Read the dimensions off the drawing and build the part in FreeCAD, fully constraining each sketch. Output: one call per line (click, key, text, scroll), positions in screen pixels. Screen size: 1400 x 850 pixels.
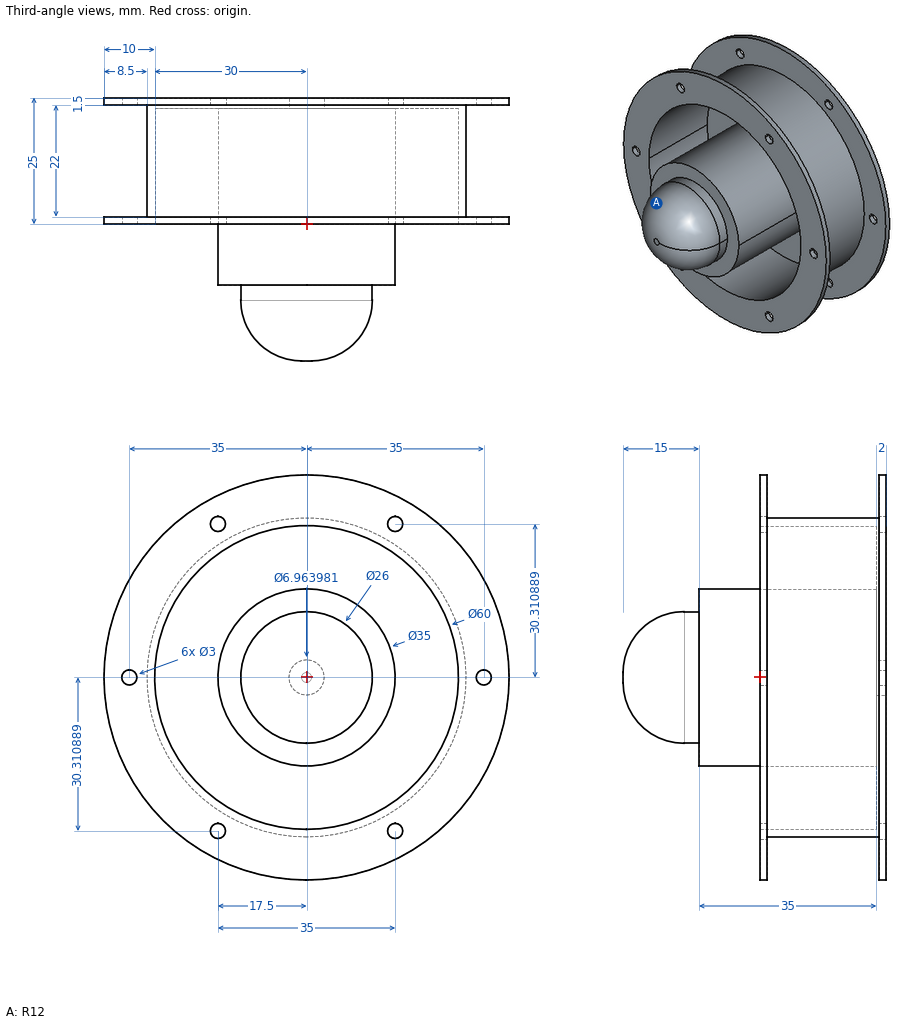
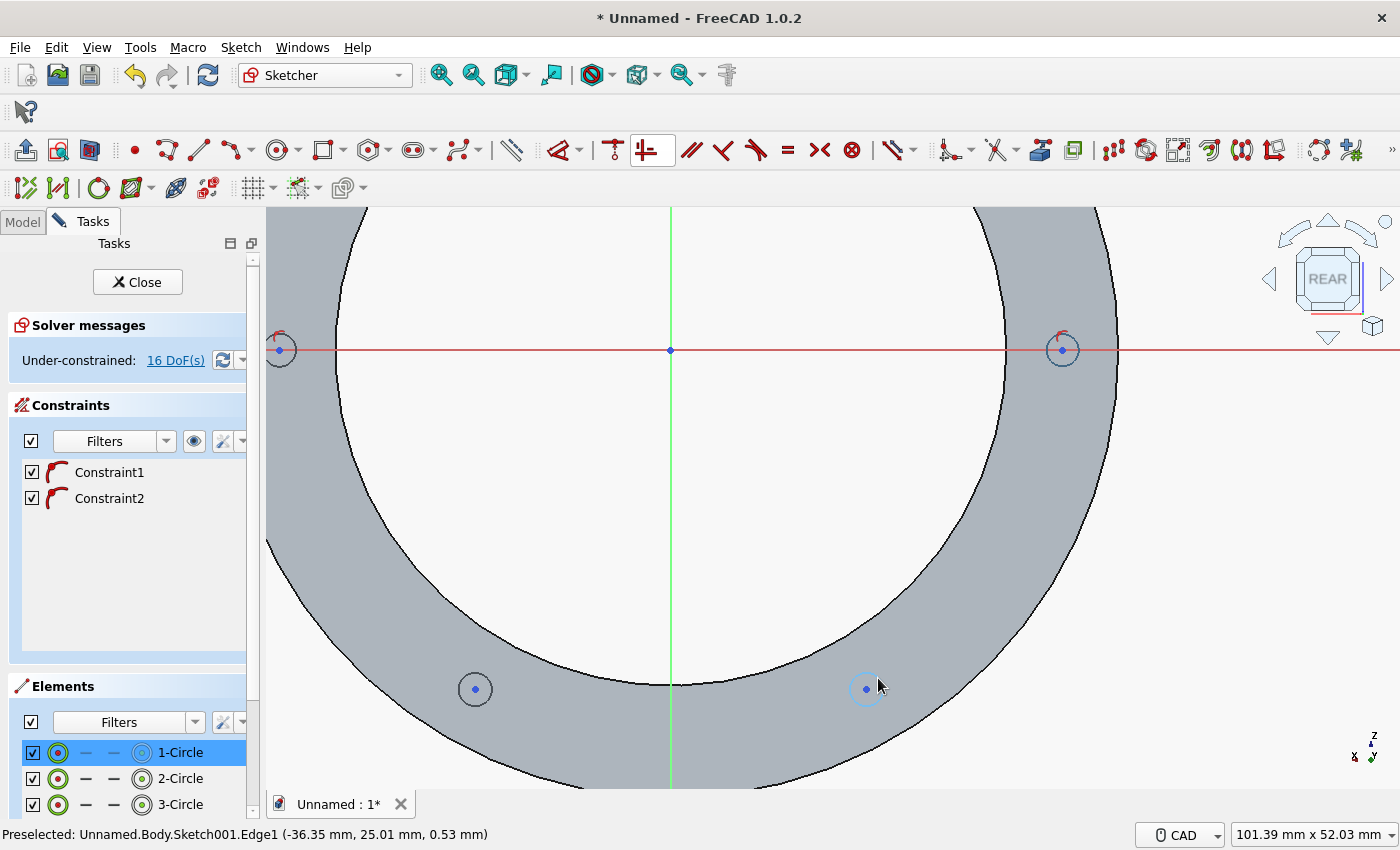
click(878, 678)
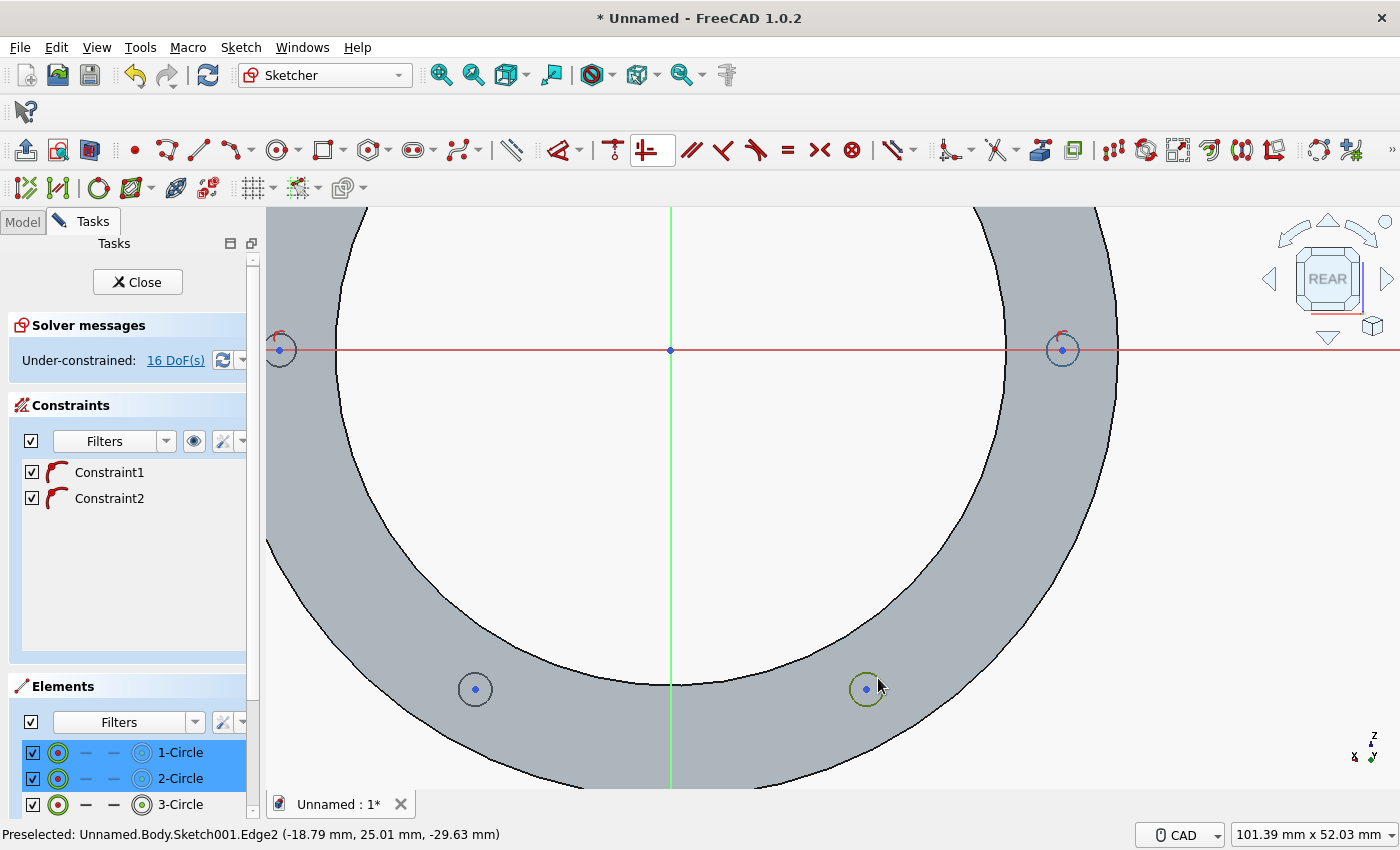
click(487, 678)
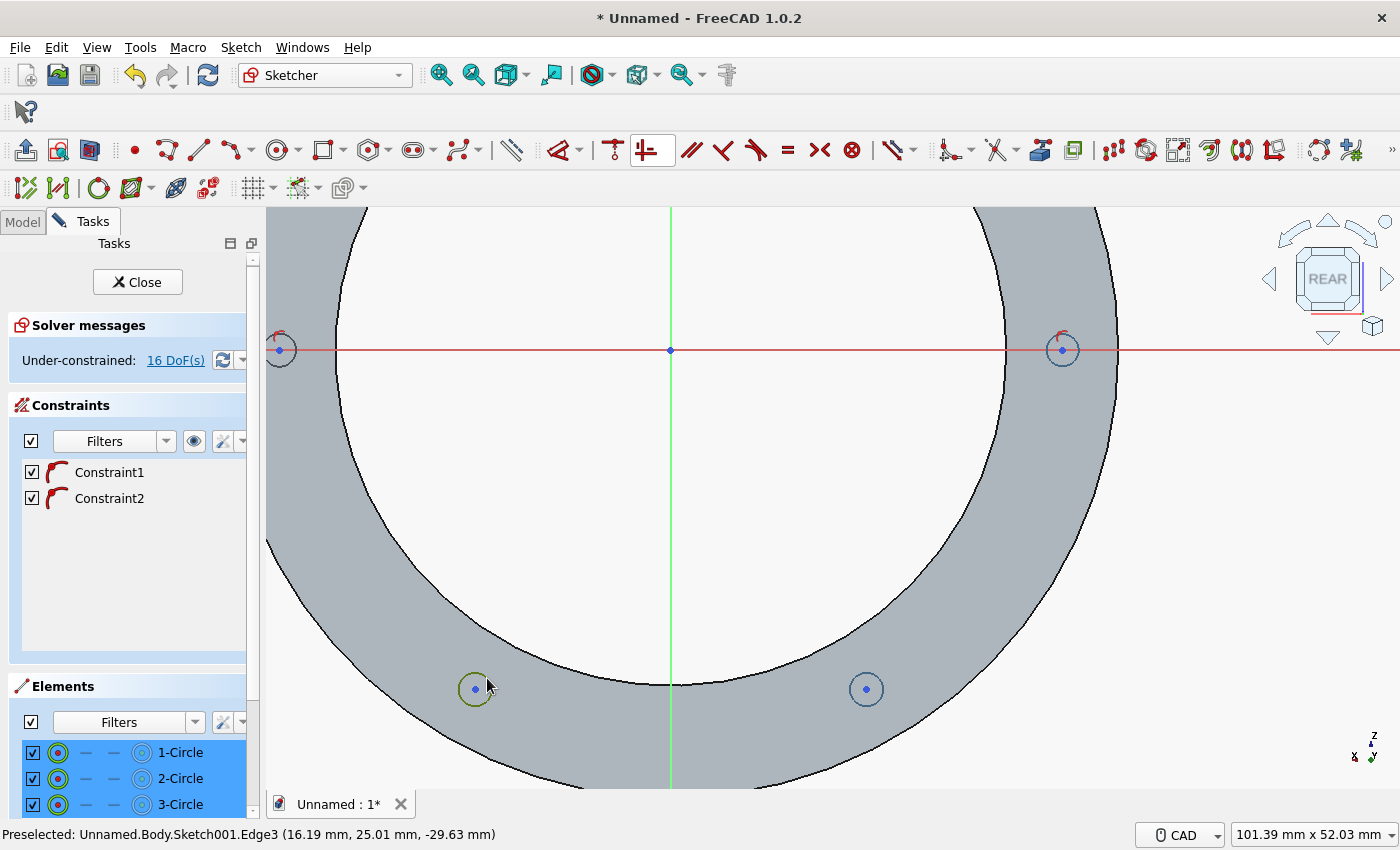
click(296, 351)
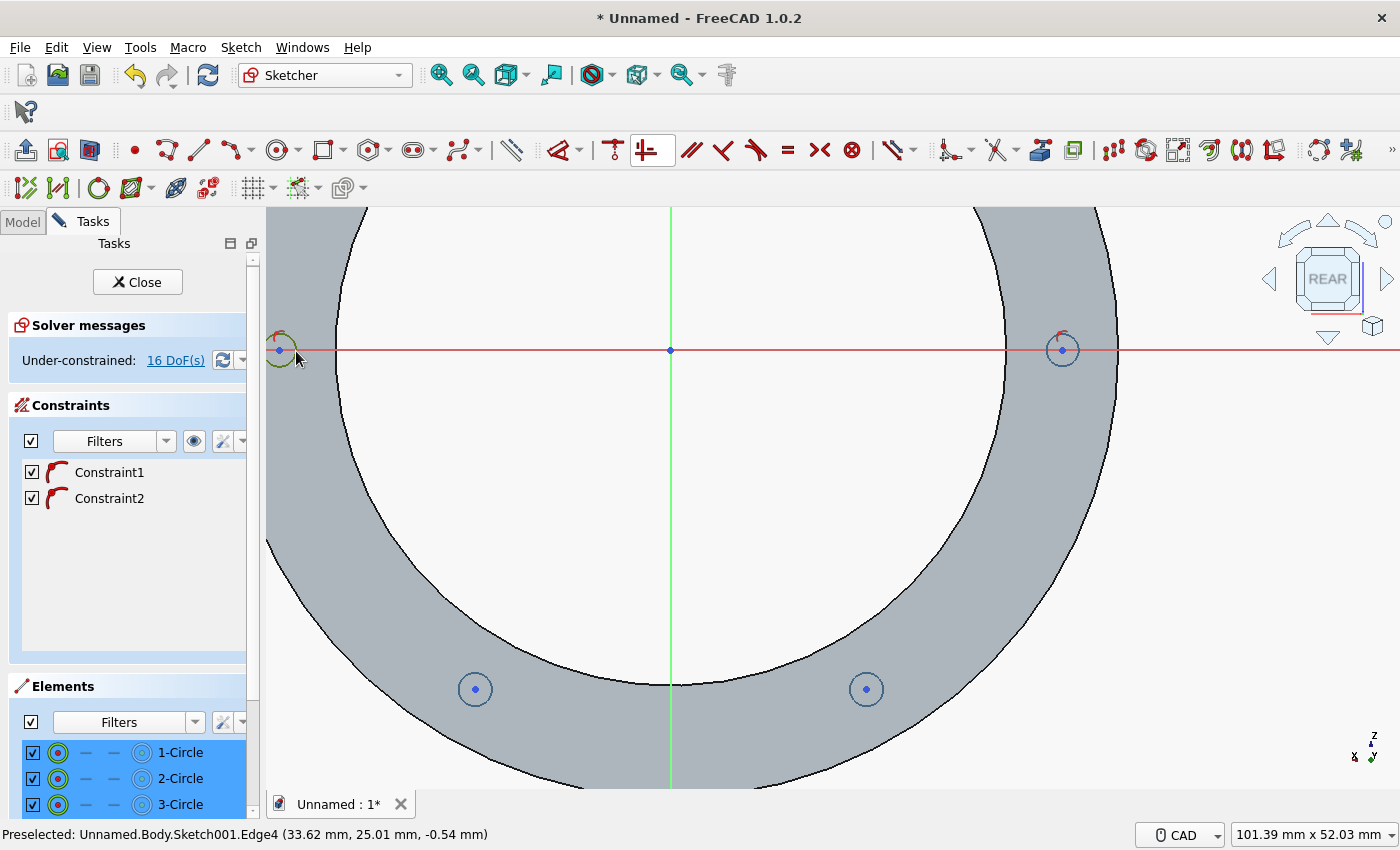
scroll(878, 678, down, 3)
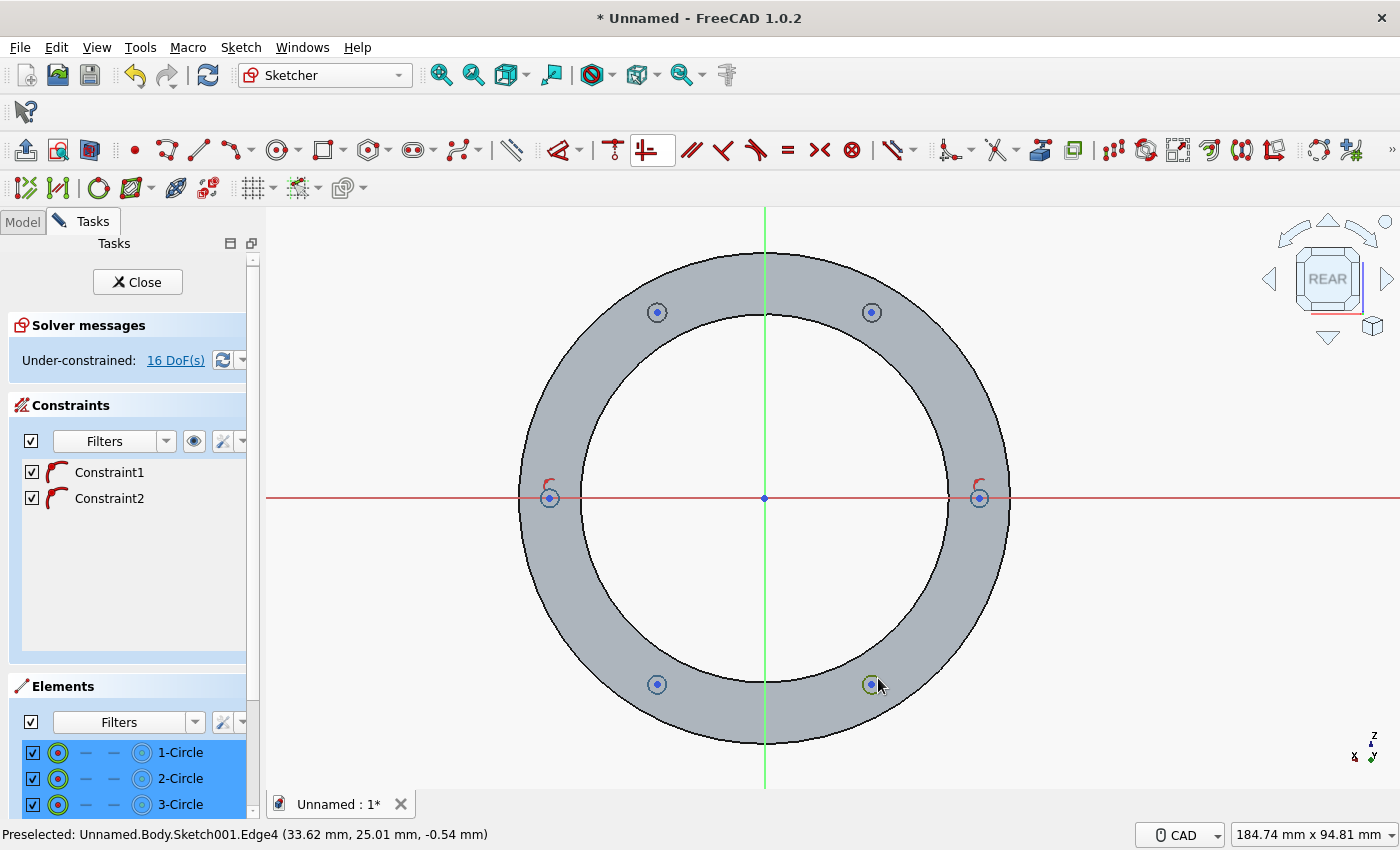
scroll(664, 306, up, 2)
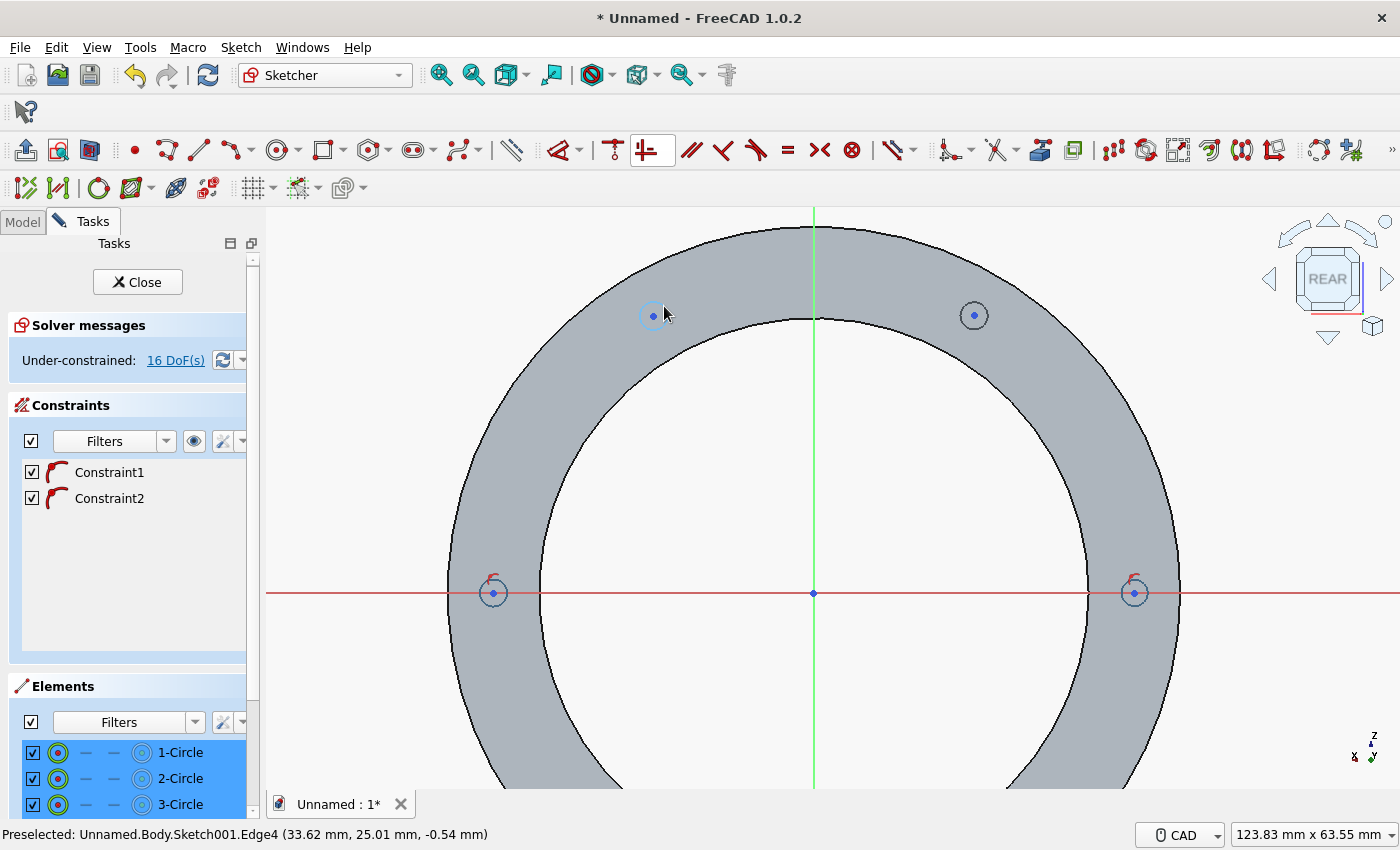
click(664, 306)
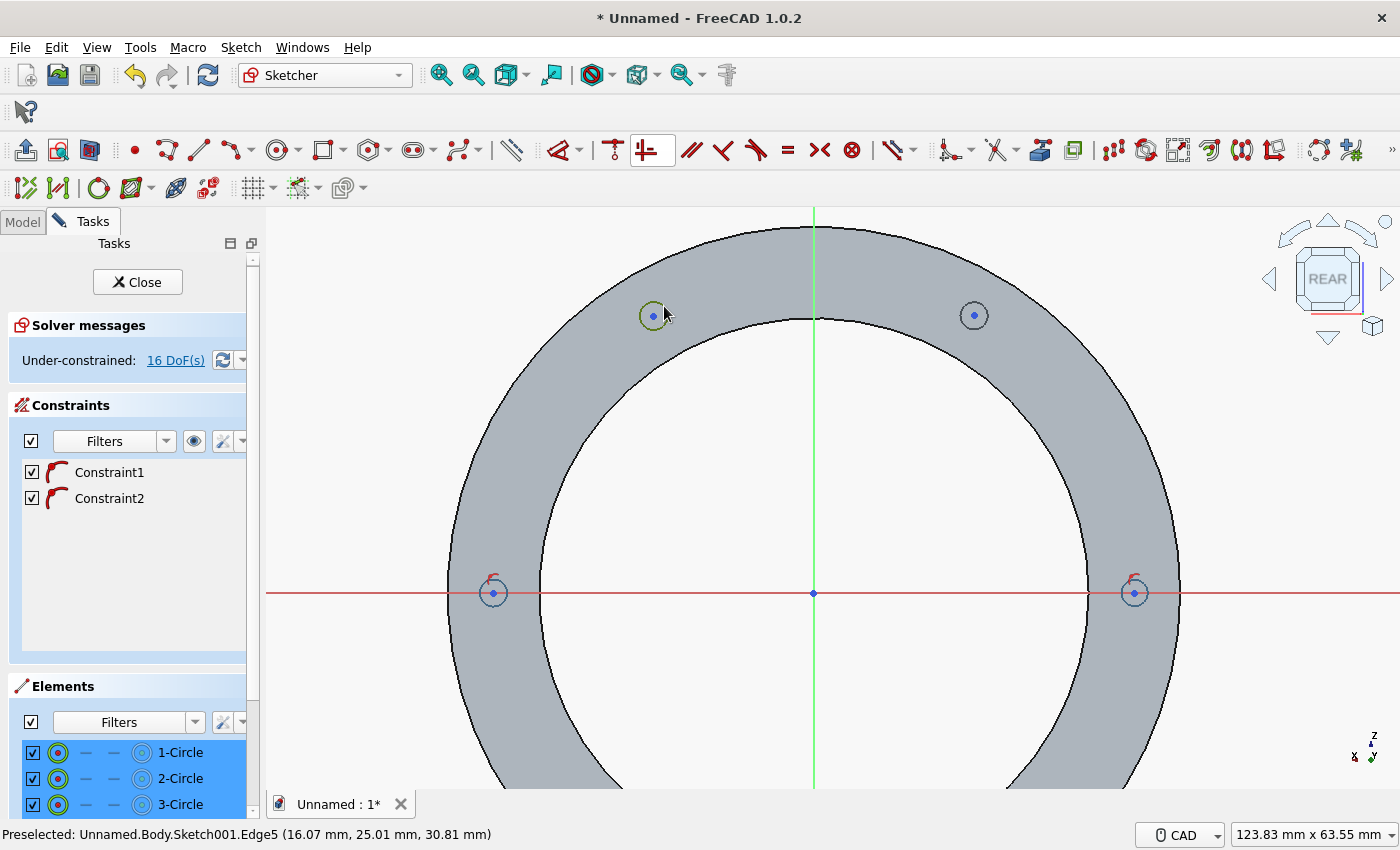
click(984, 306)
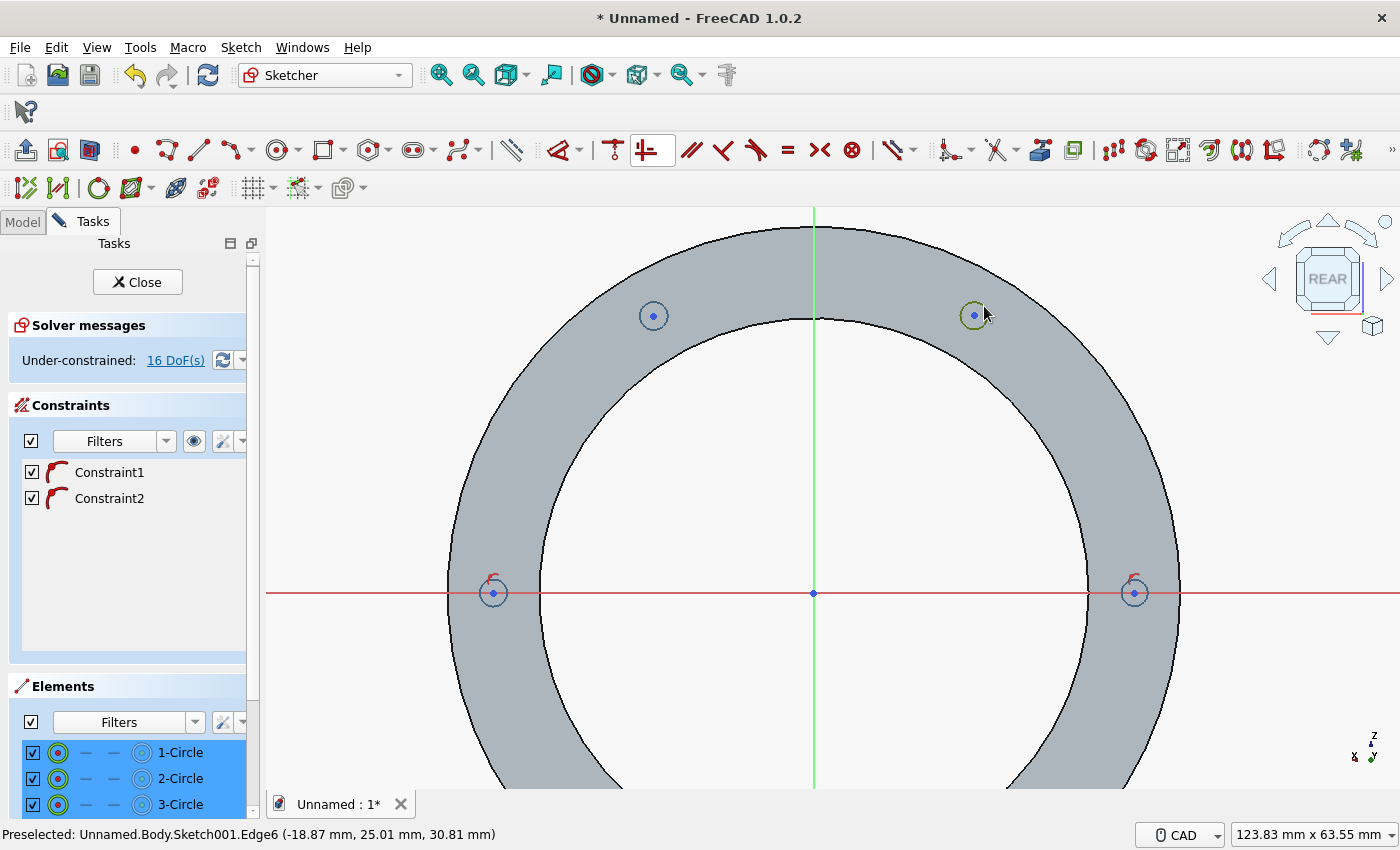
click(788, 150)